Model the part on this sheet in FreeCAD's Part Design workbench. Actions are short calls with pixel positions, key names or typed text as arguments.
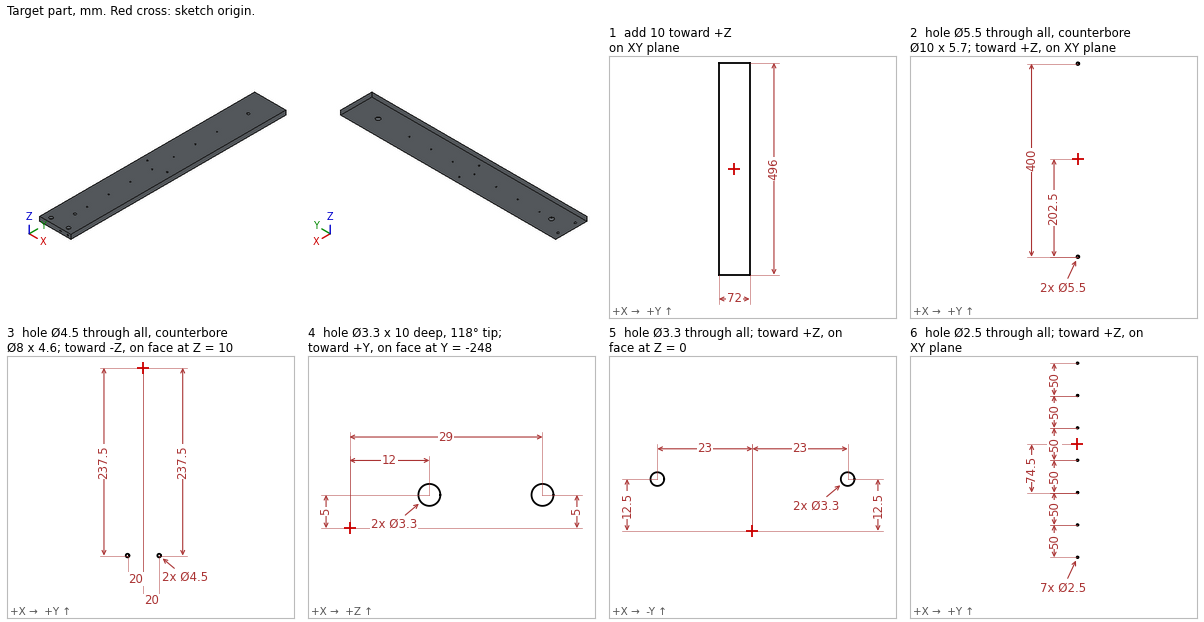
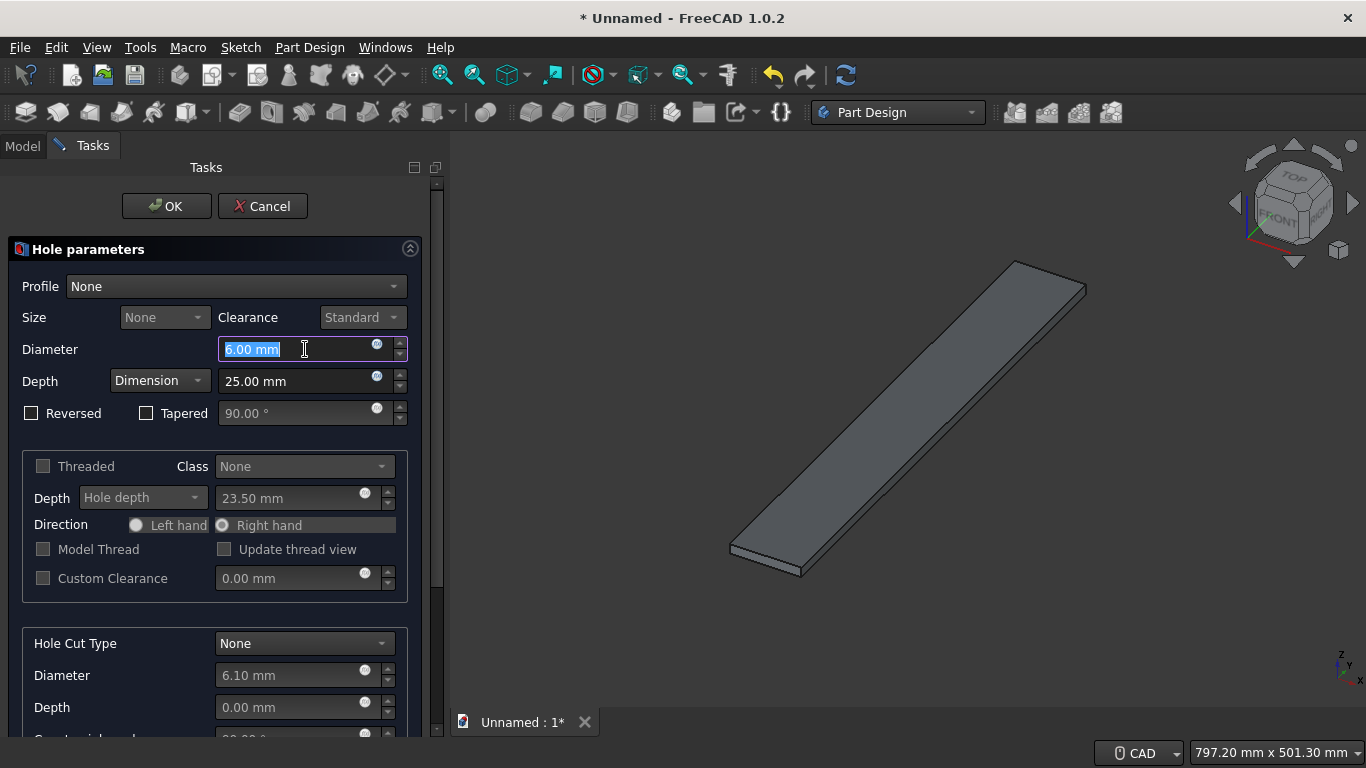
text(5.5)
key(Tab)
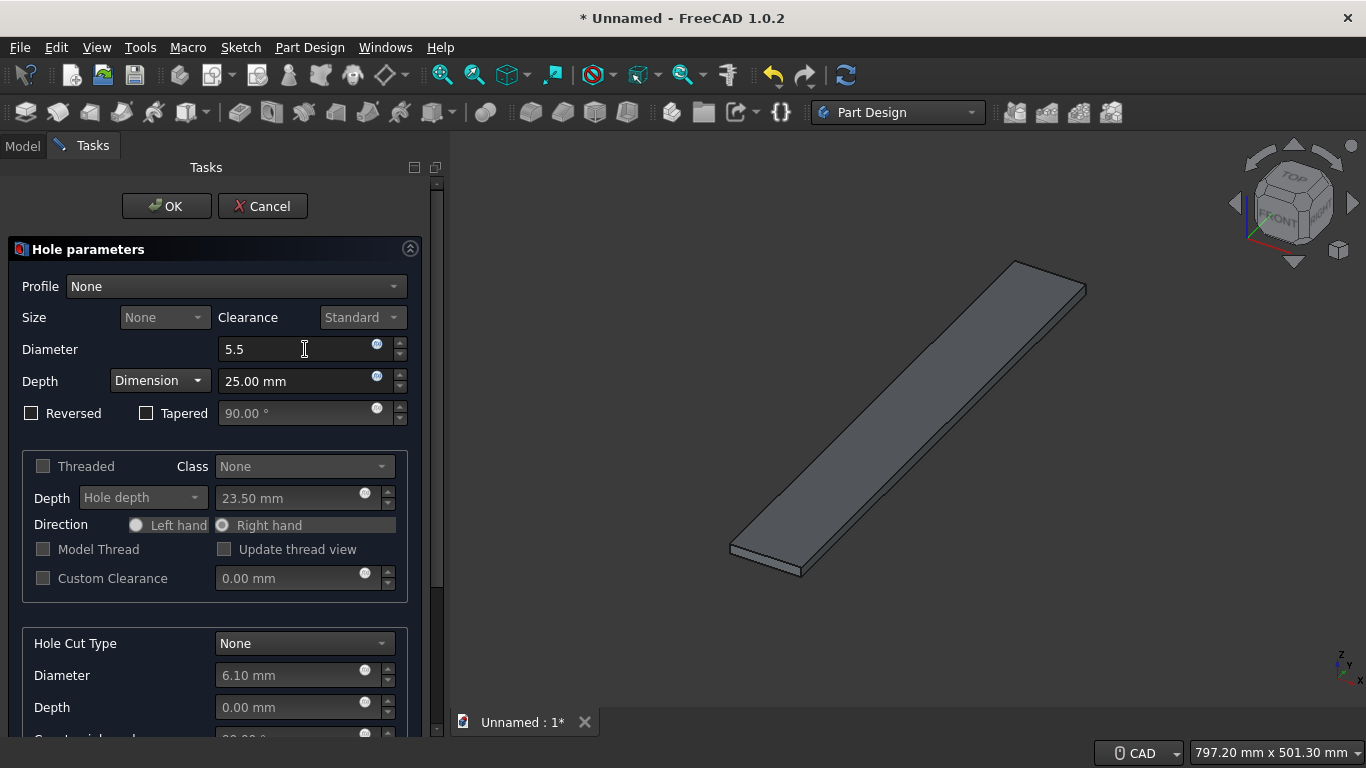
click(161, 380)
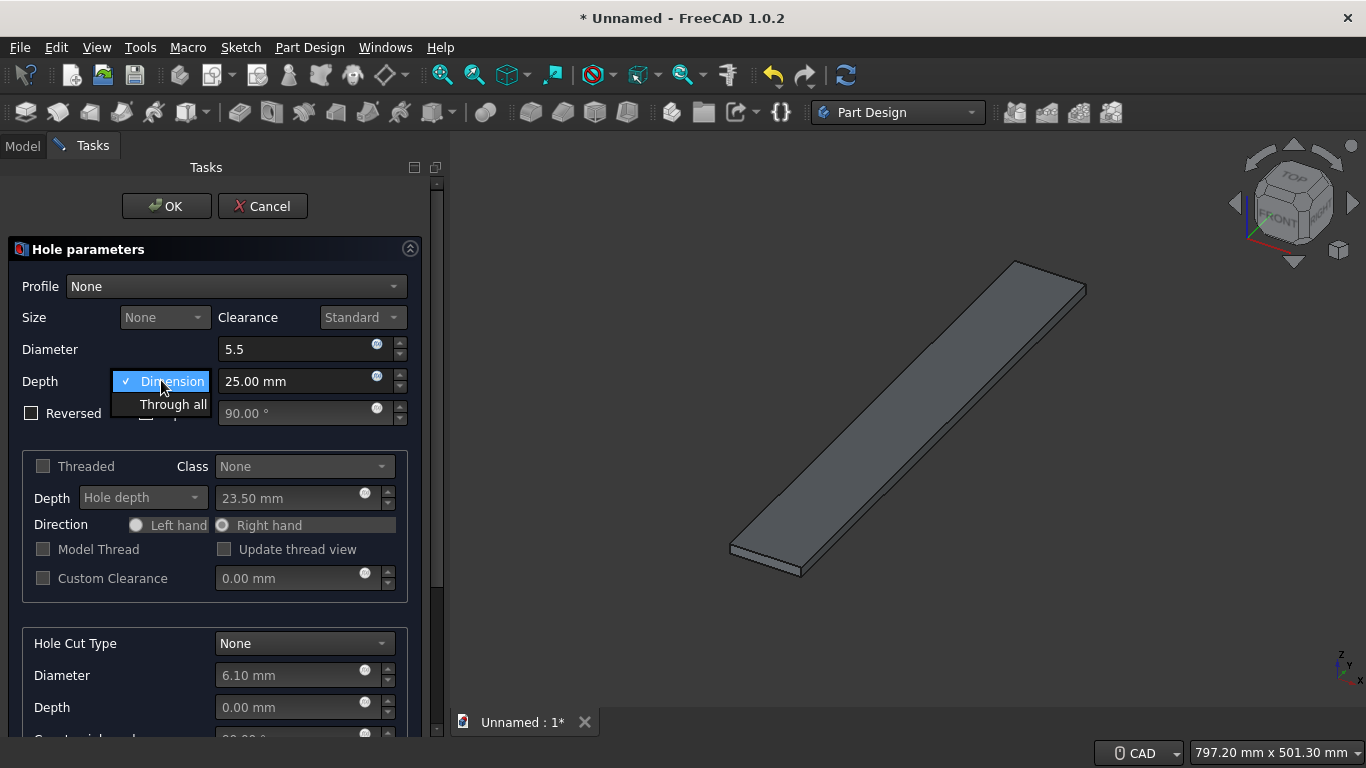
click(160, 404)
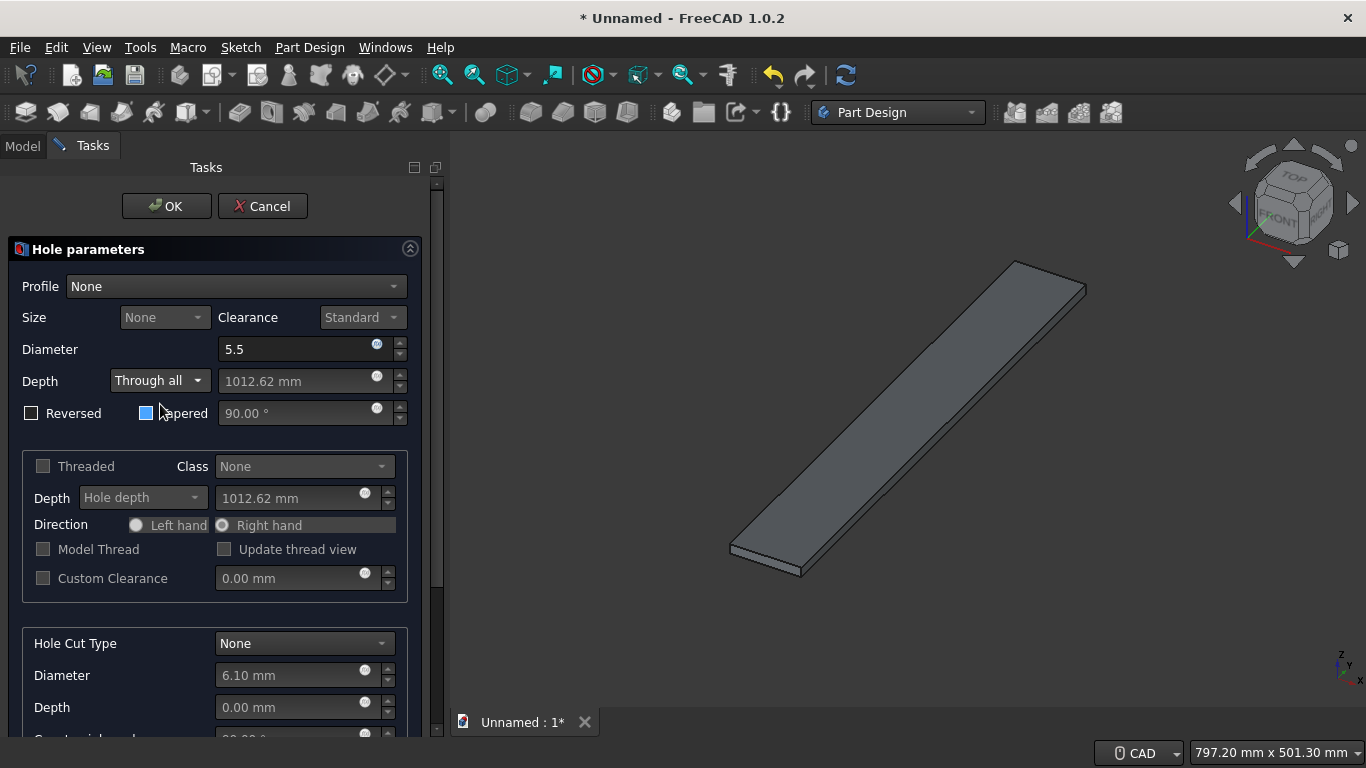
click(30, 413)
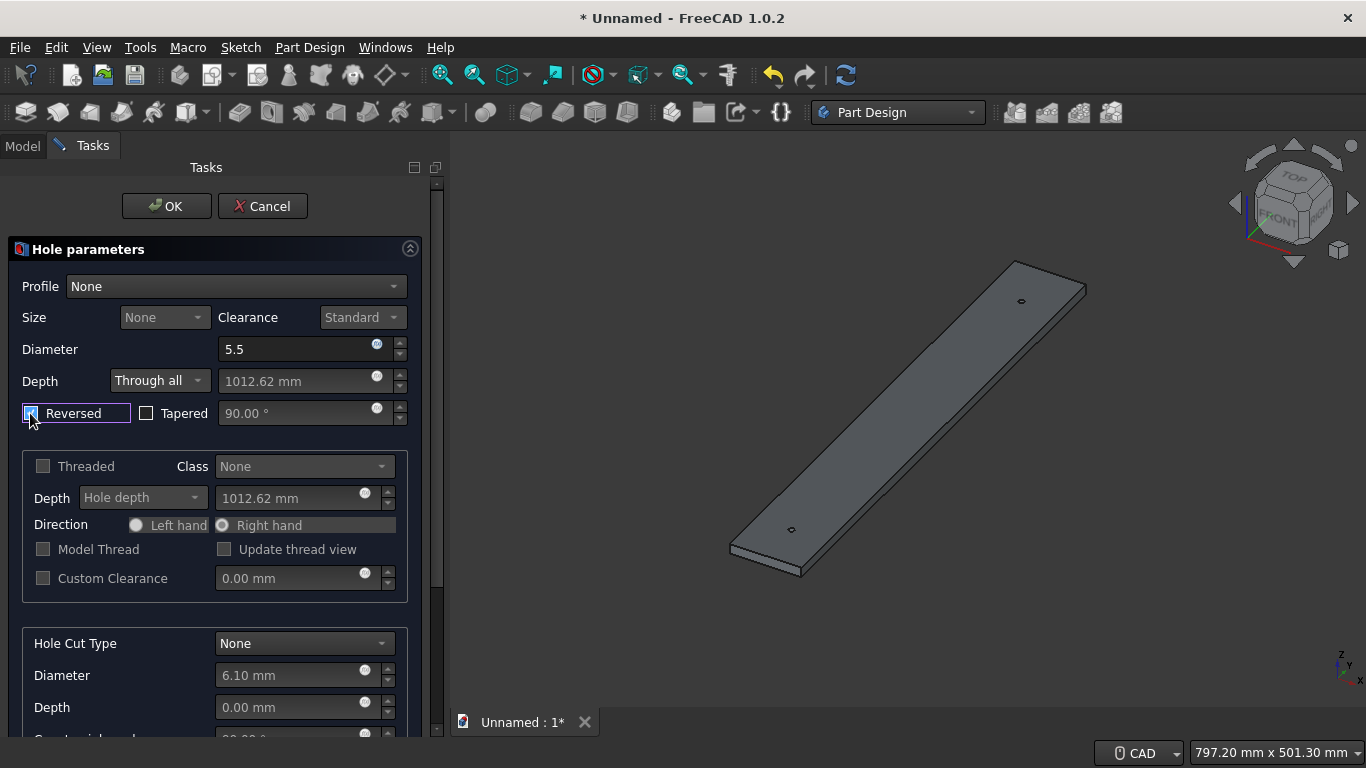
click(306, 644)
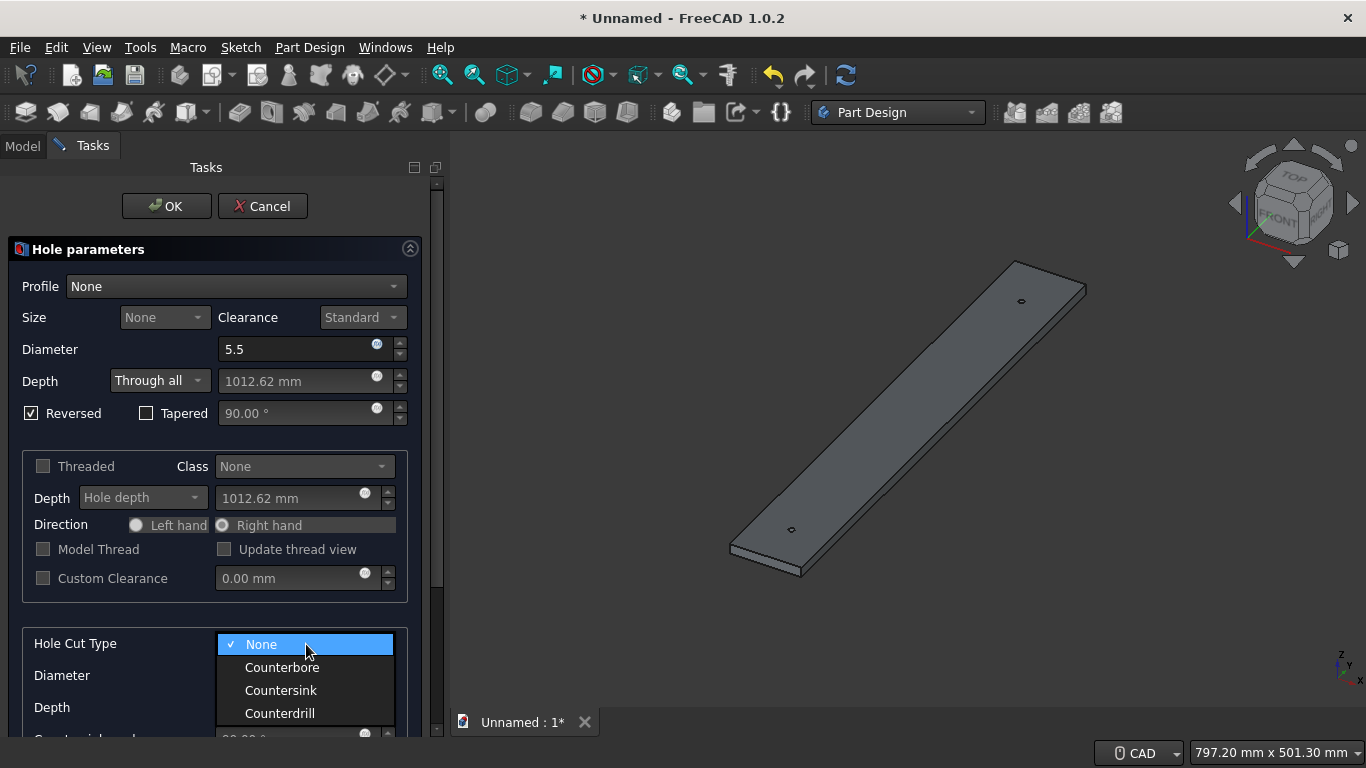
click(304, 668)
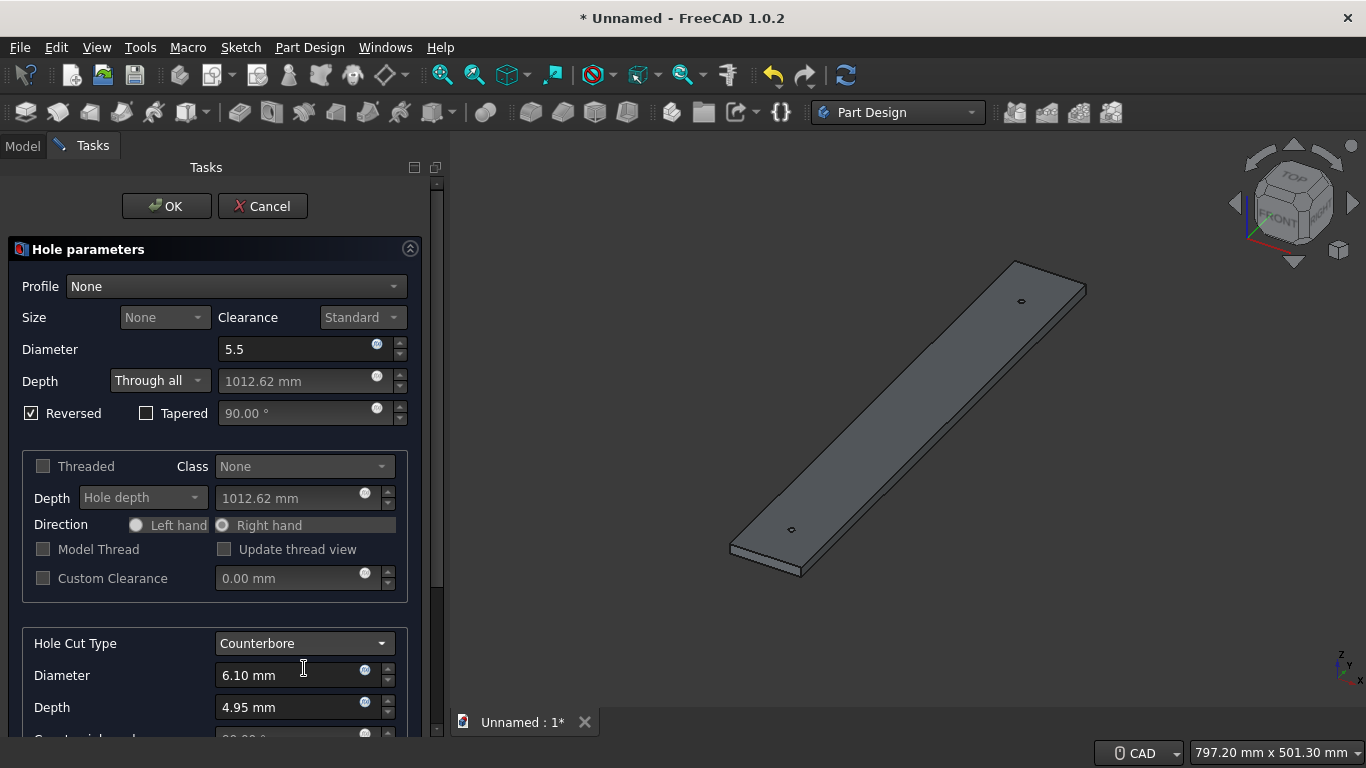
triple_click(298, 675)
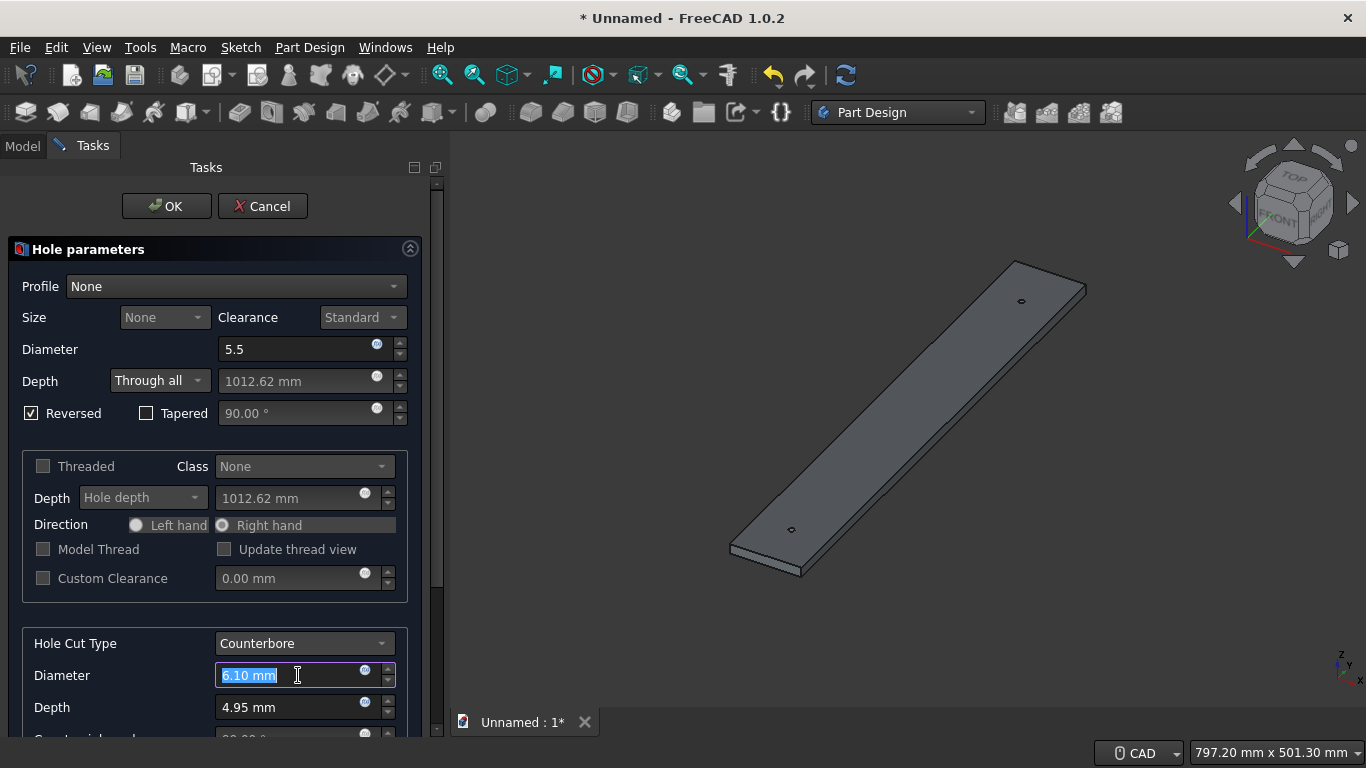
text(10)
key(Tab)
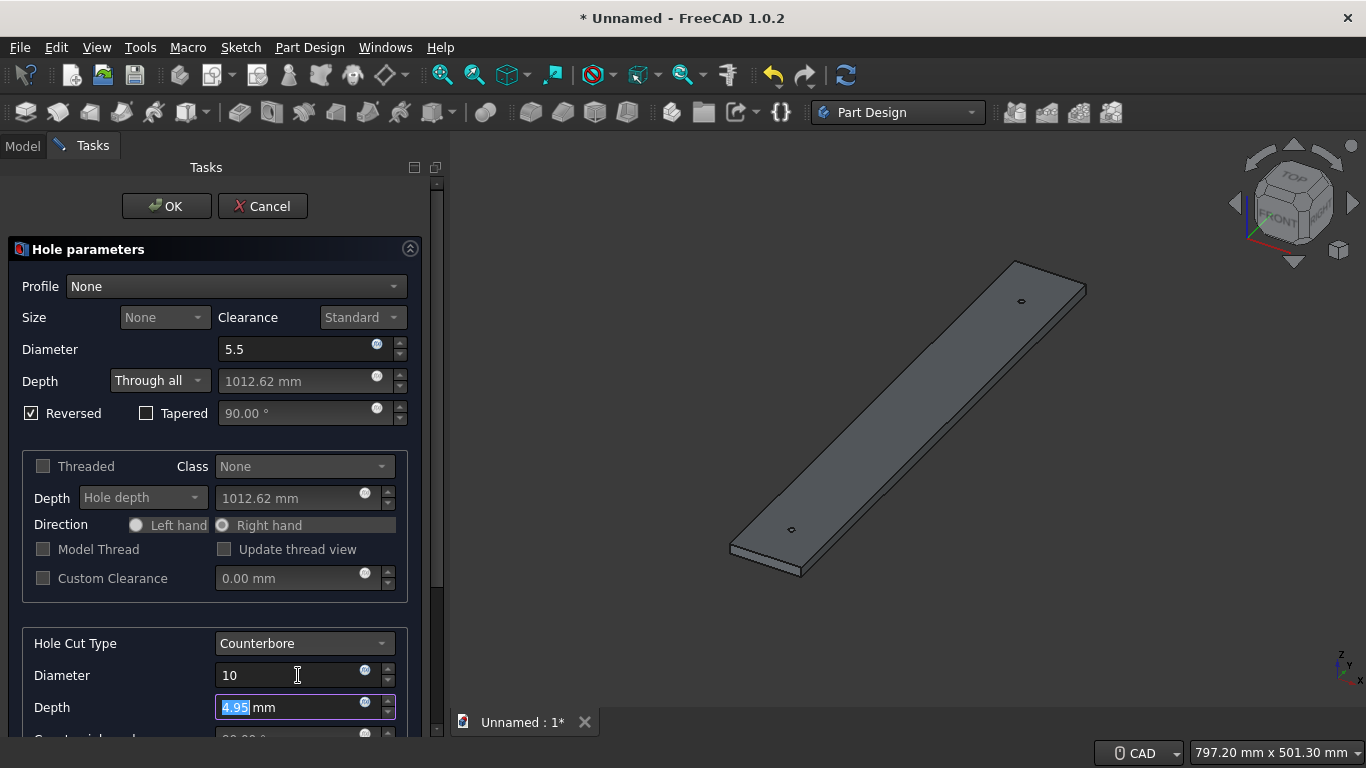
text(5.7)
key(Tab)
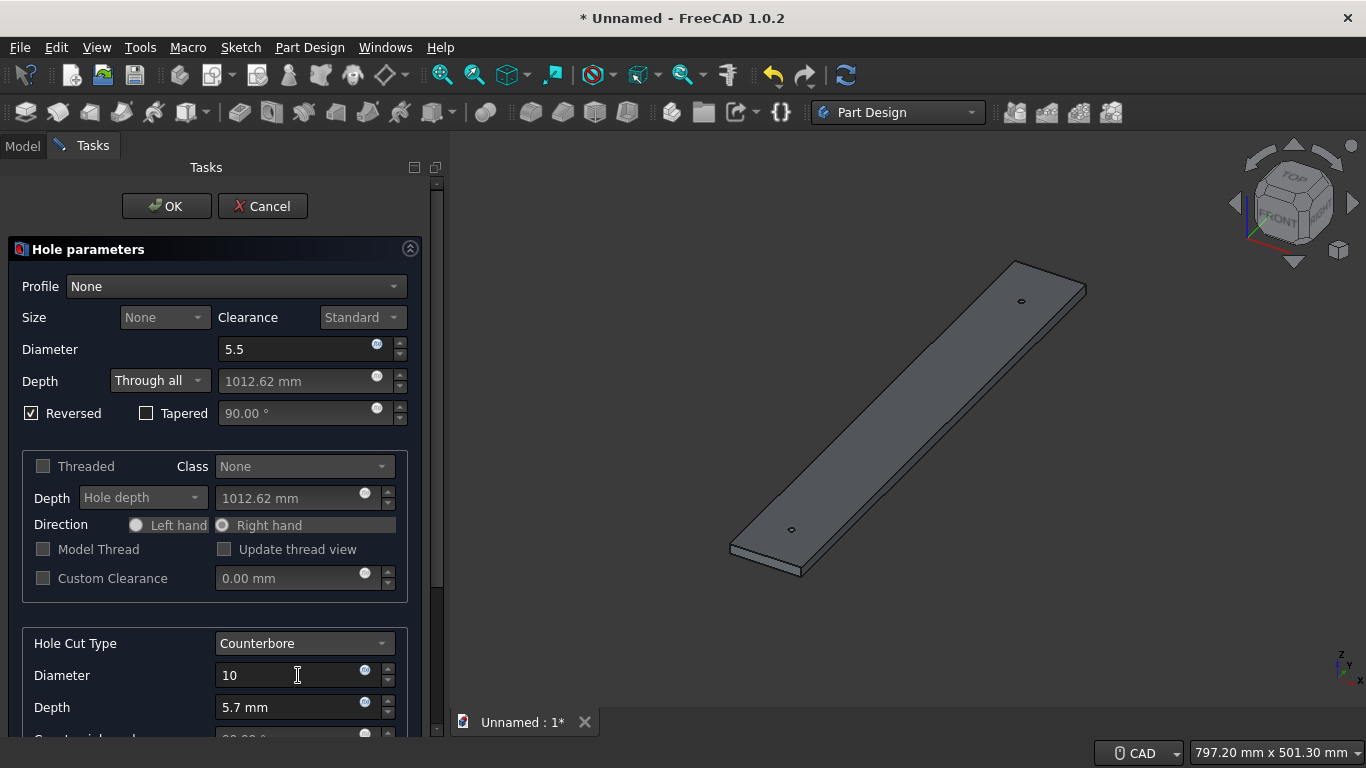
click(167, 206)